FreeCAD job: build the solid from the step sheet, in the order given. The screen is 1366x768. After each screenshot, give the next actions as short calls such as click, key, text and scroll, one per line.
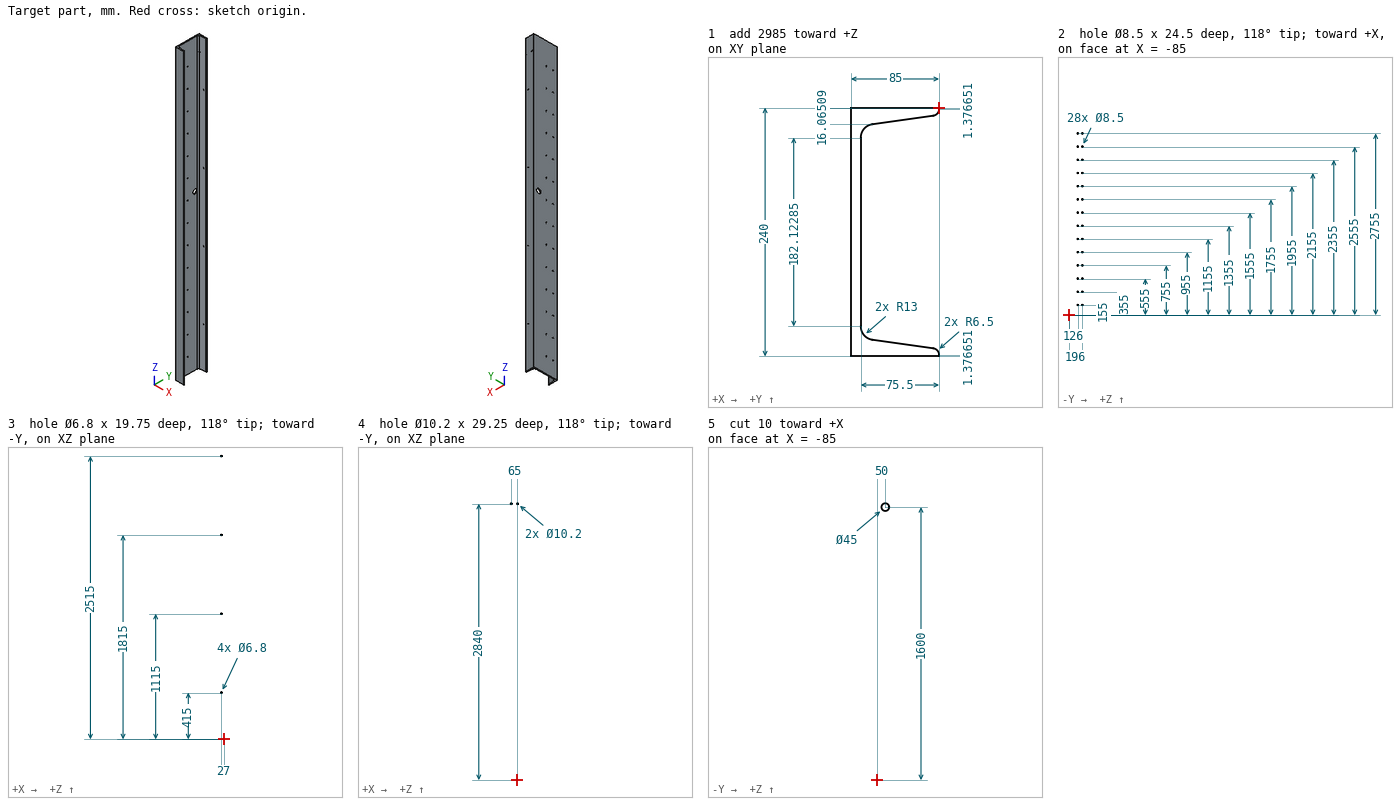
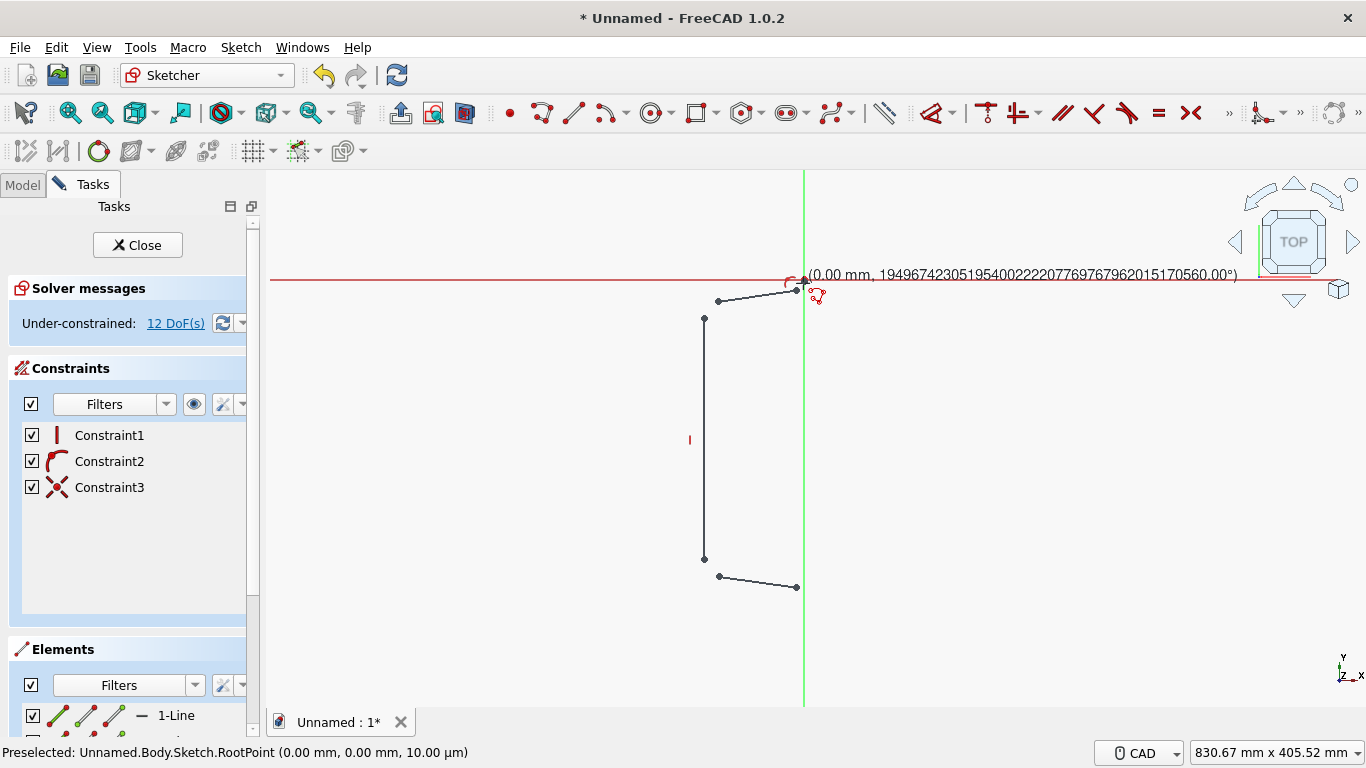
click(692, 289)
click(692, 598)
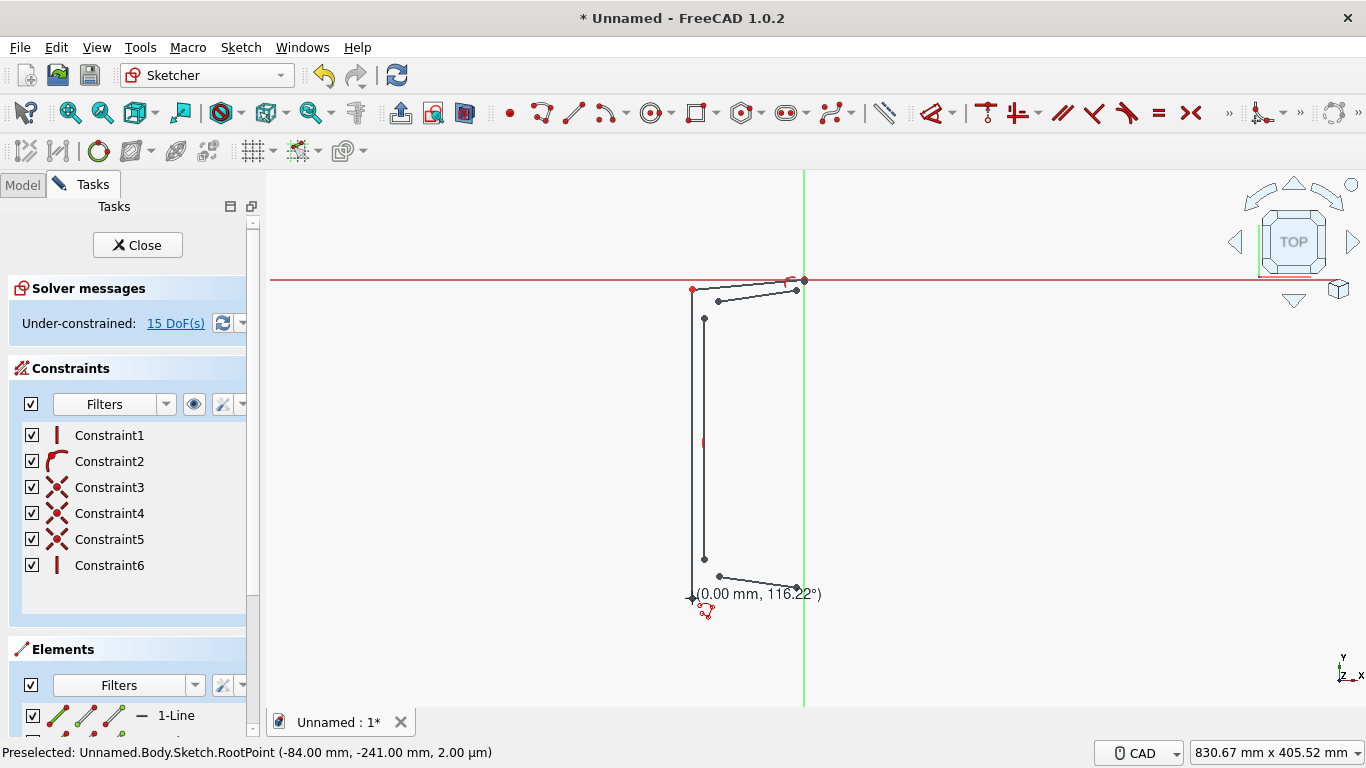
scroll(804, 598, up, 2)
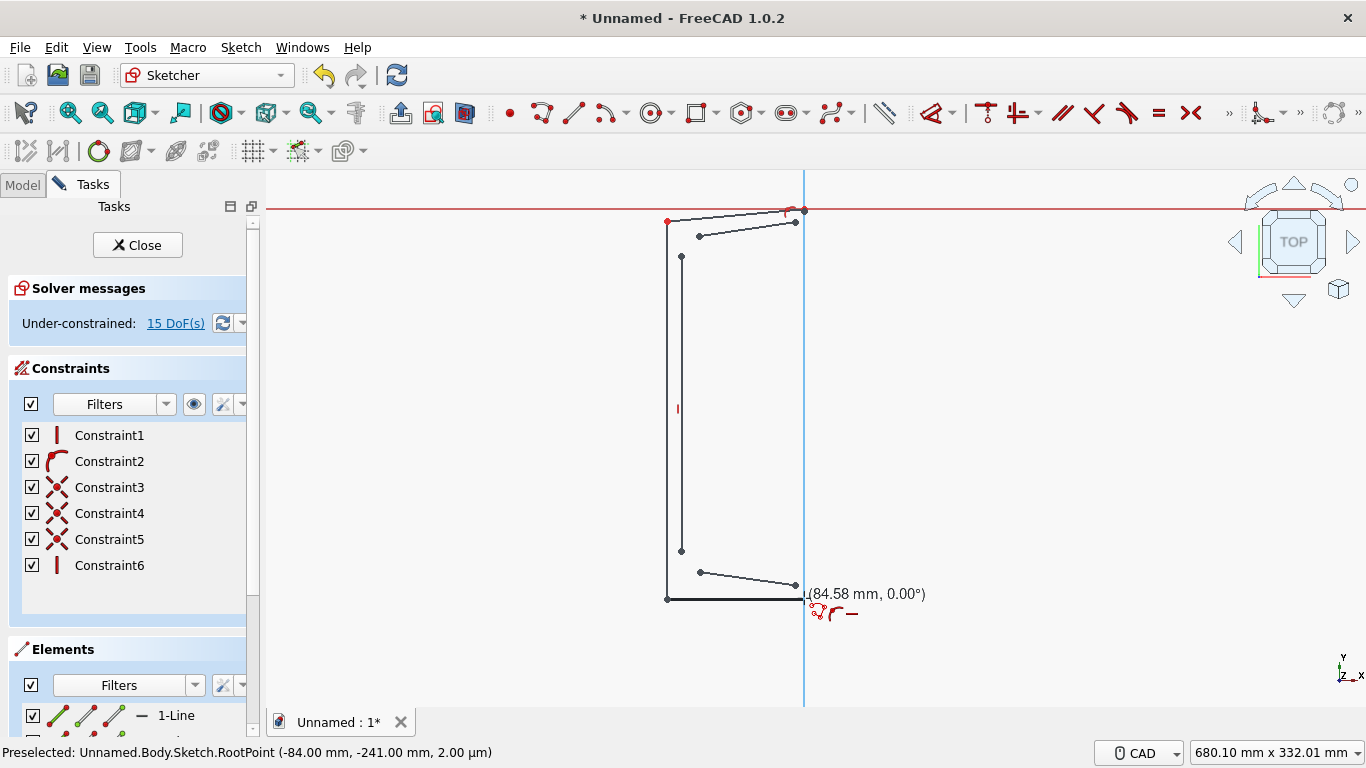
click(804, 598)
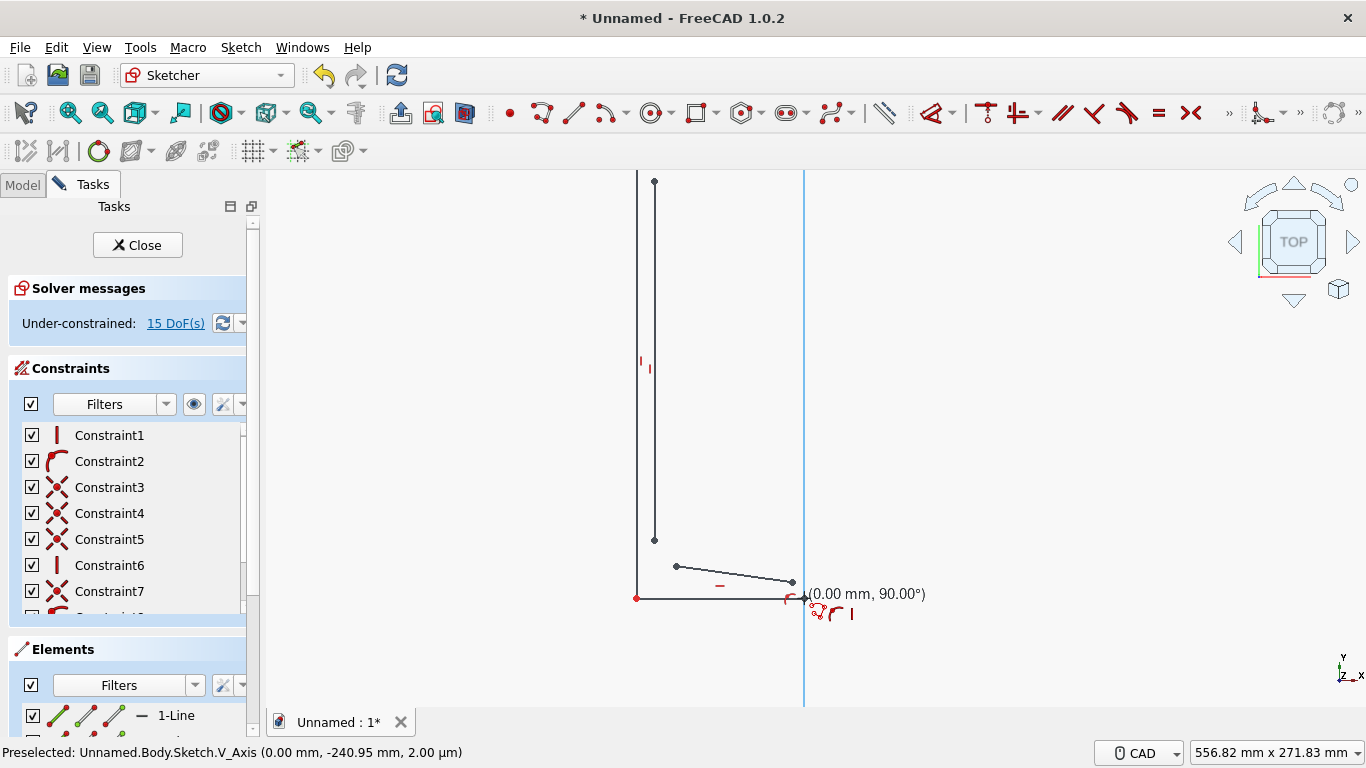
scroll(804, 594, up, 9)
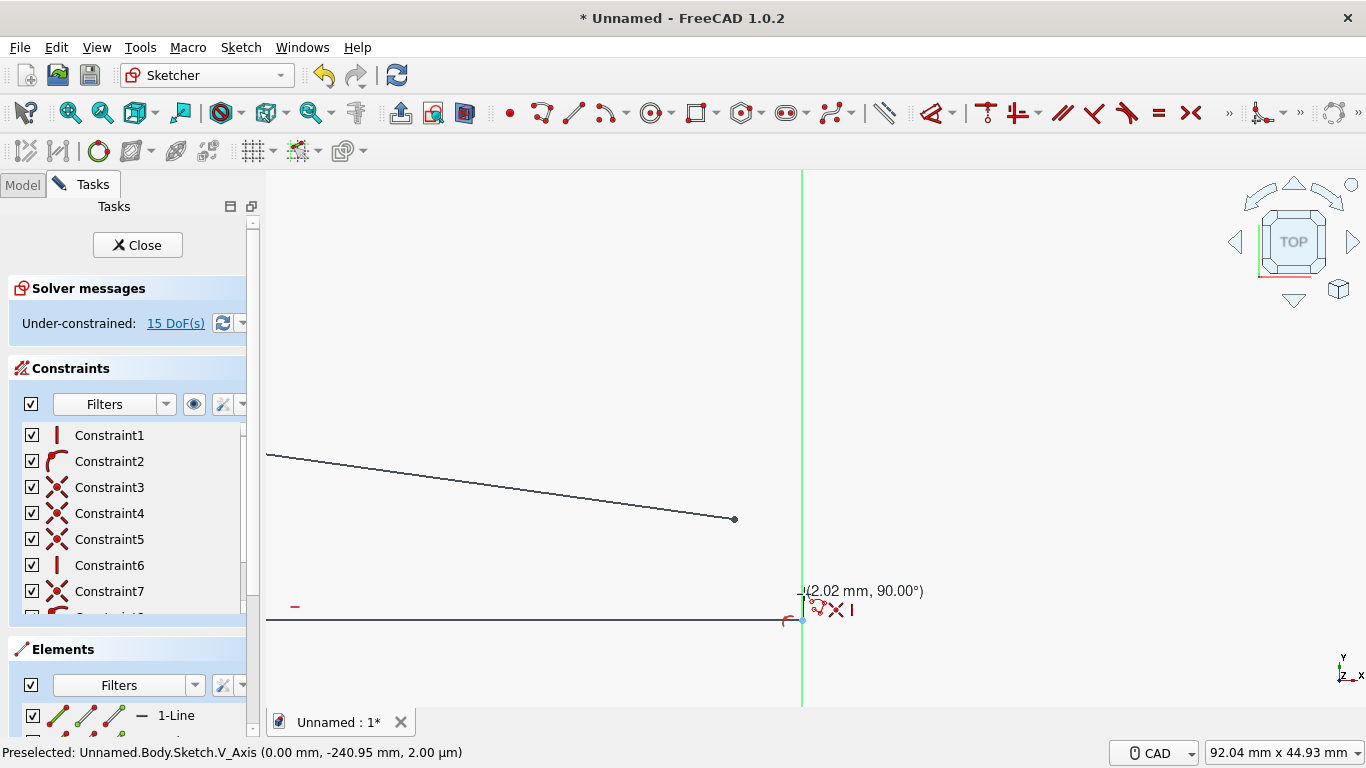
click(793, 592)
right_click(793, 592)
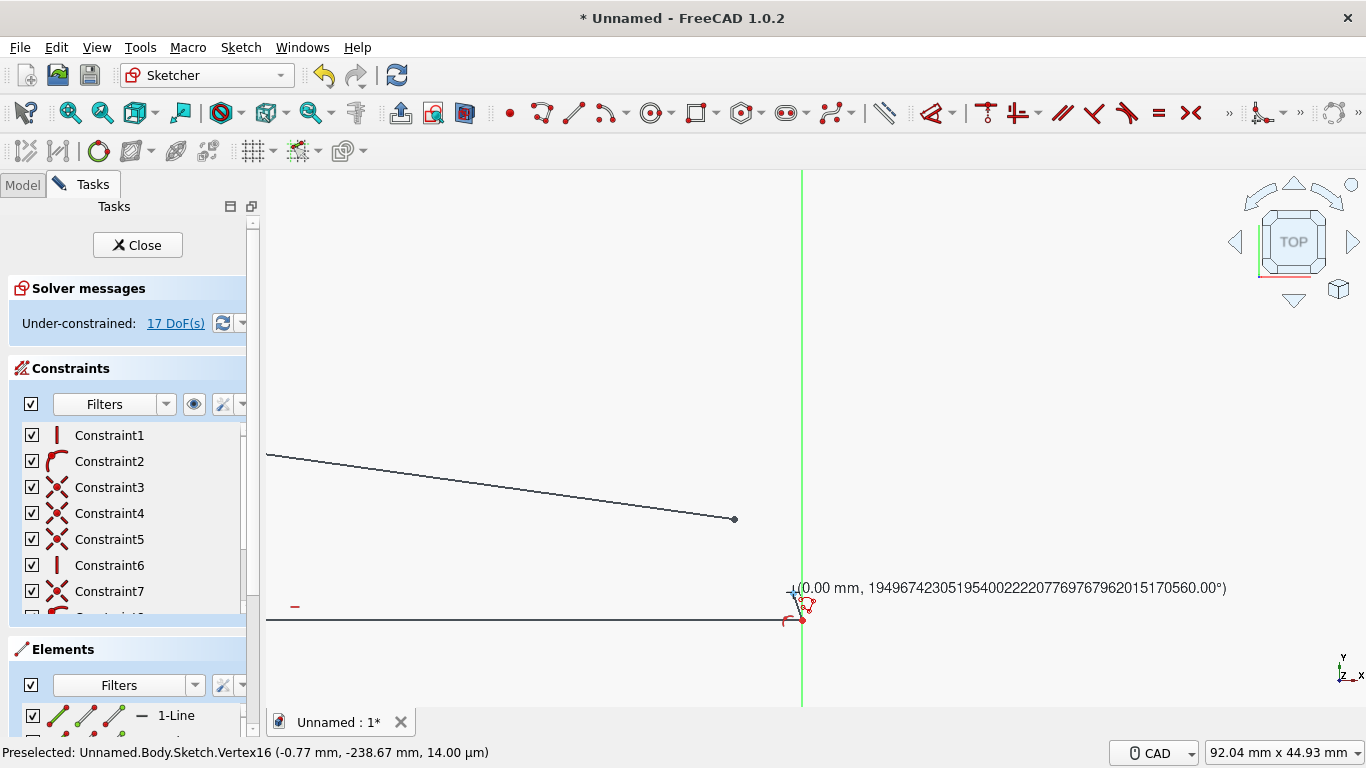
key(g)
key(3)
key(a)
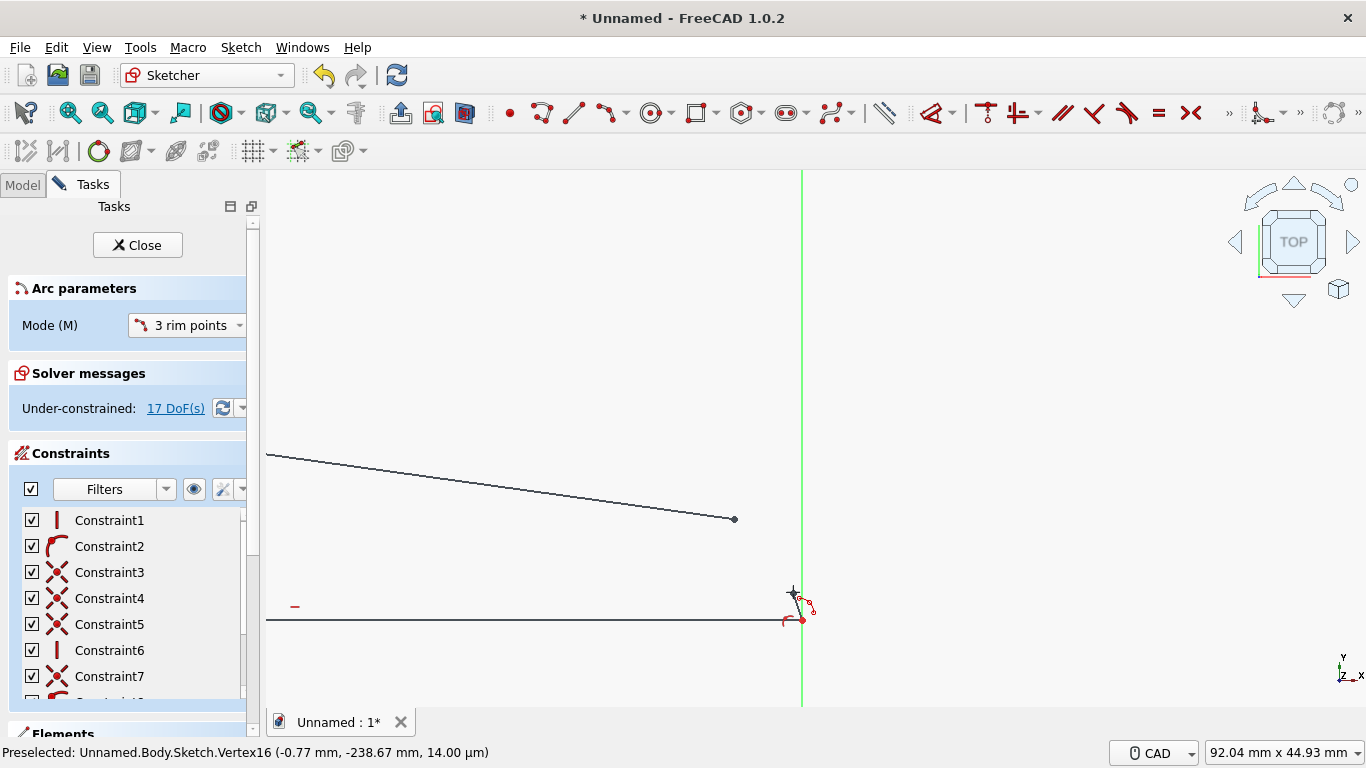
scroll(804, 596, down, 11)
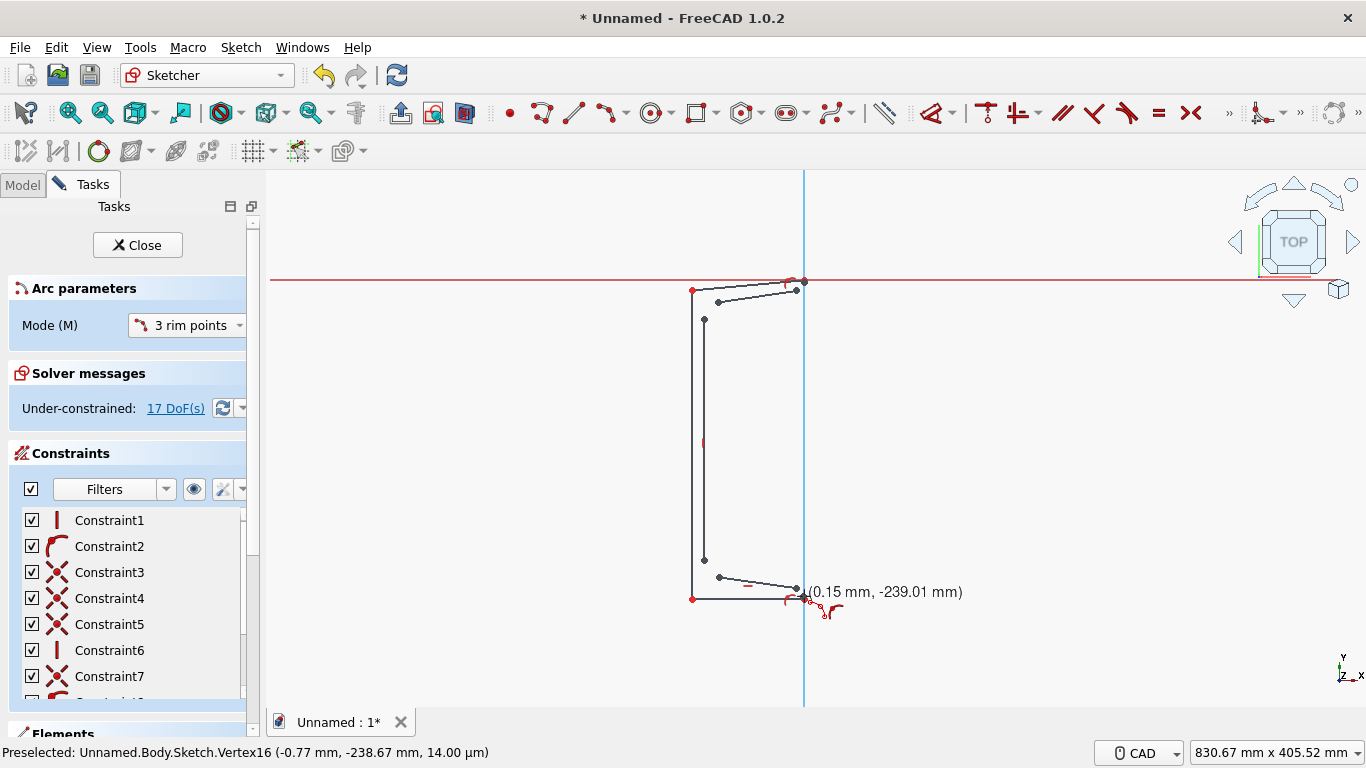
click(719, 577)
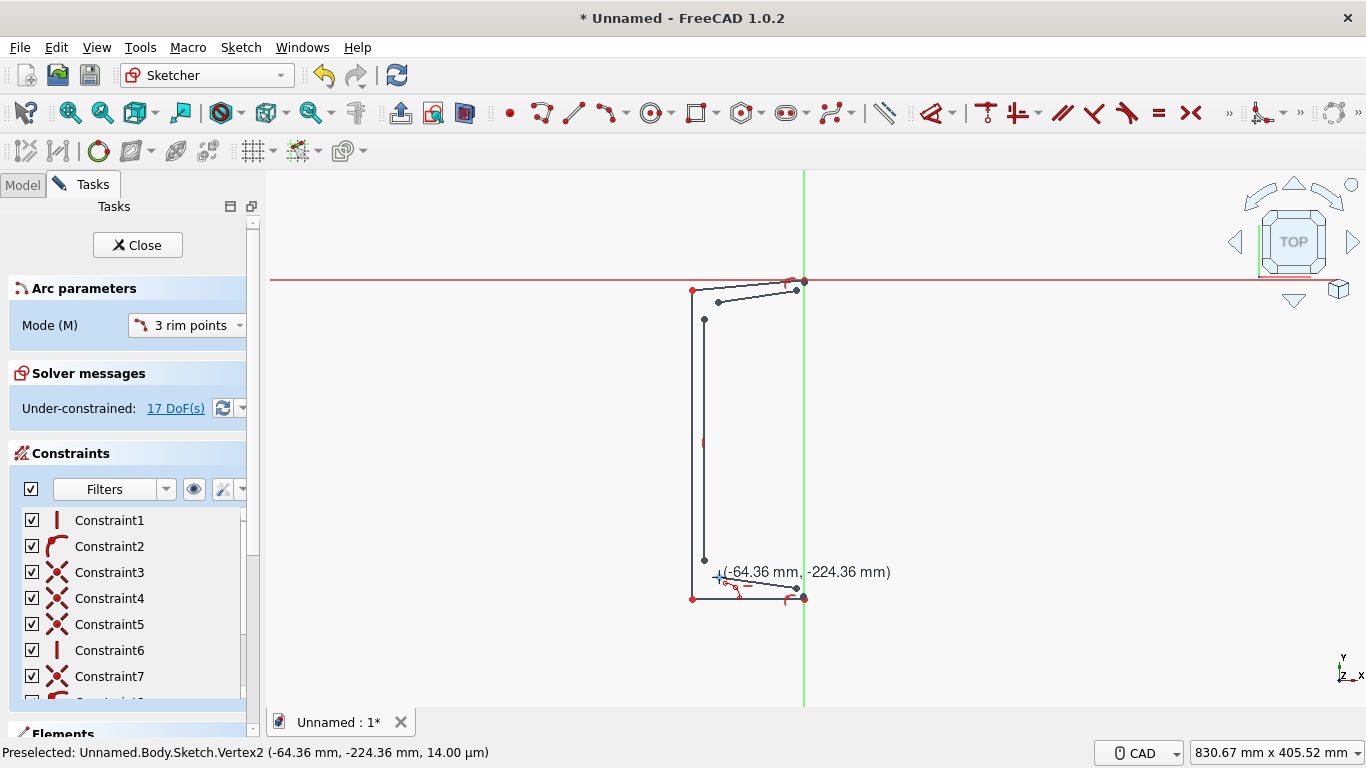
scroll(704, 560, up, 2)